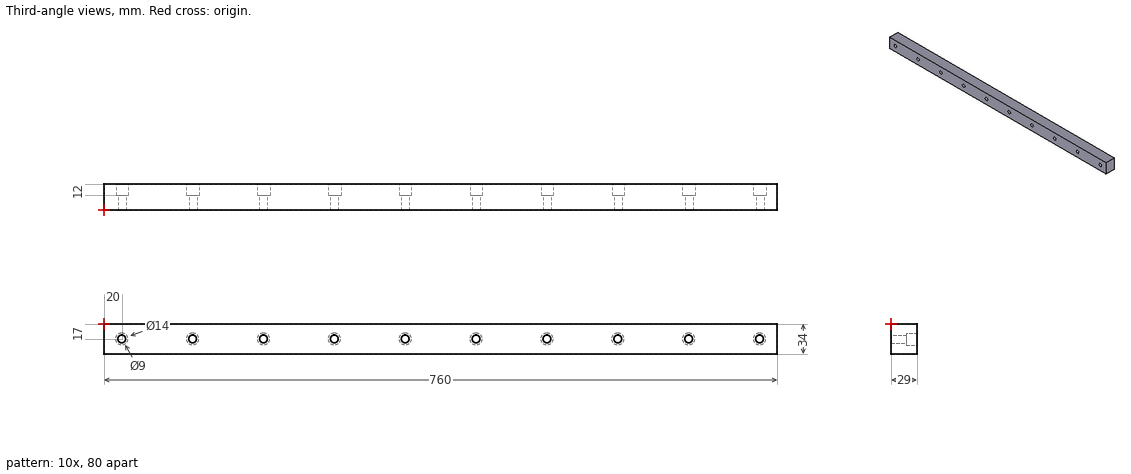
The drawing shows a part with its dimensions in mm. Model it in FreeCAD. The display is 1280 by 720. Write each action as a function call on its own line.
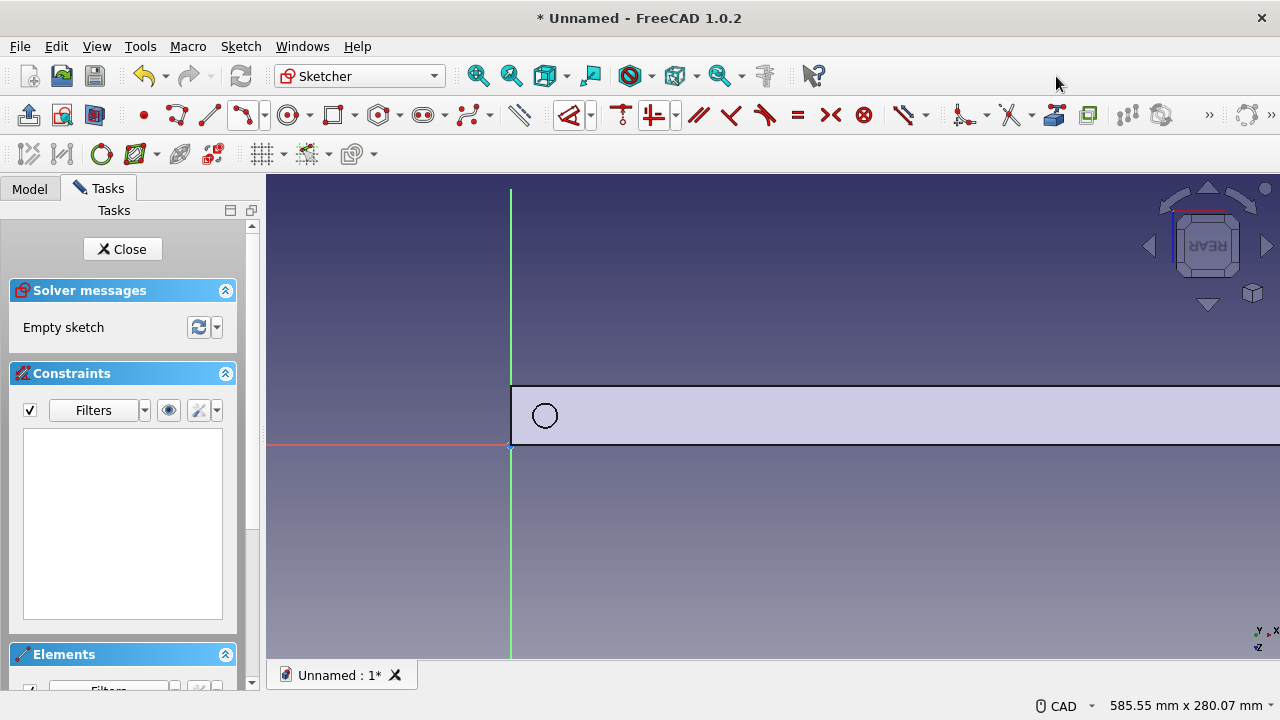
scroll(537, 416, up, 15)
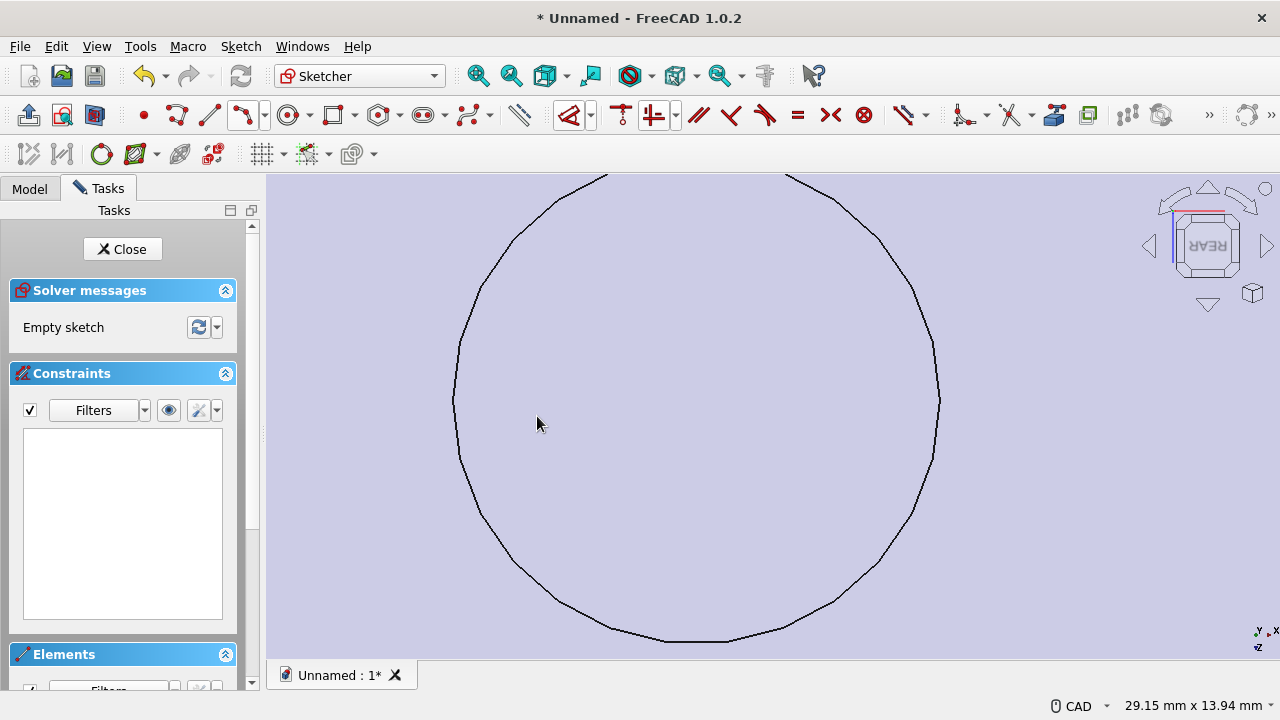
key(g)
key(c)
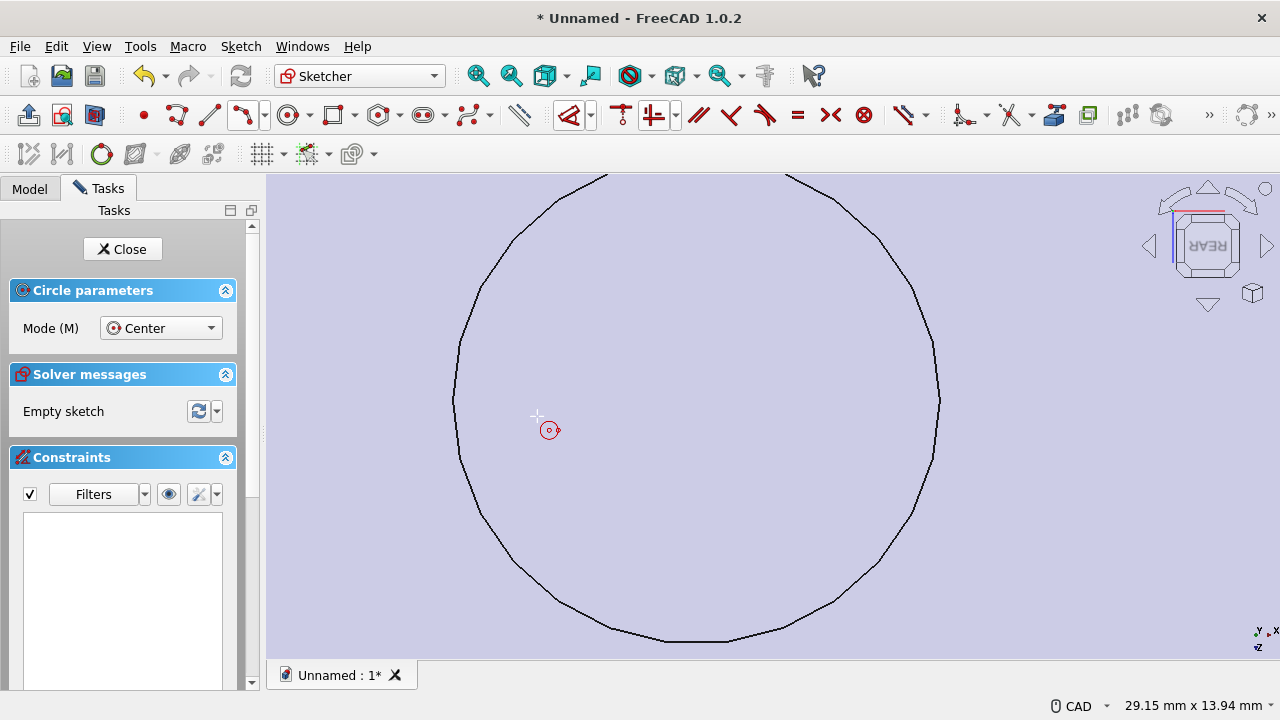
click(696, 400)
move(807, 290)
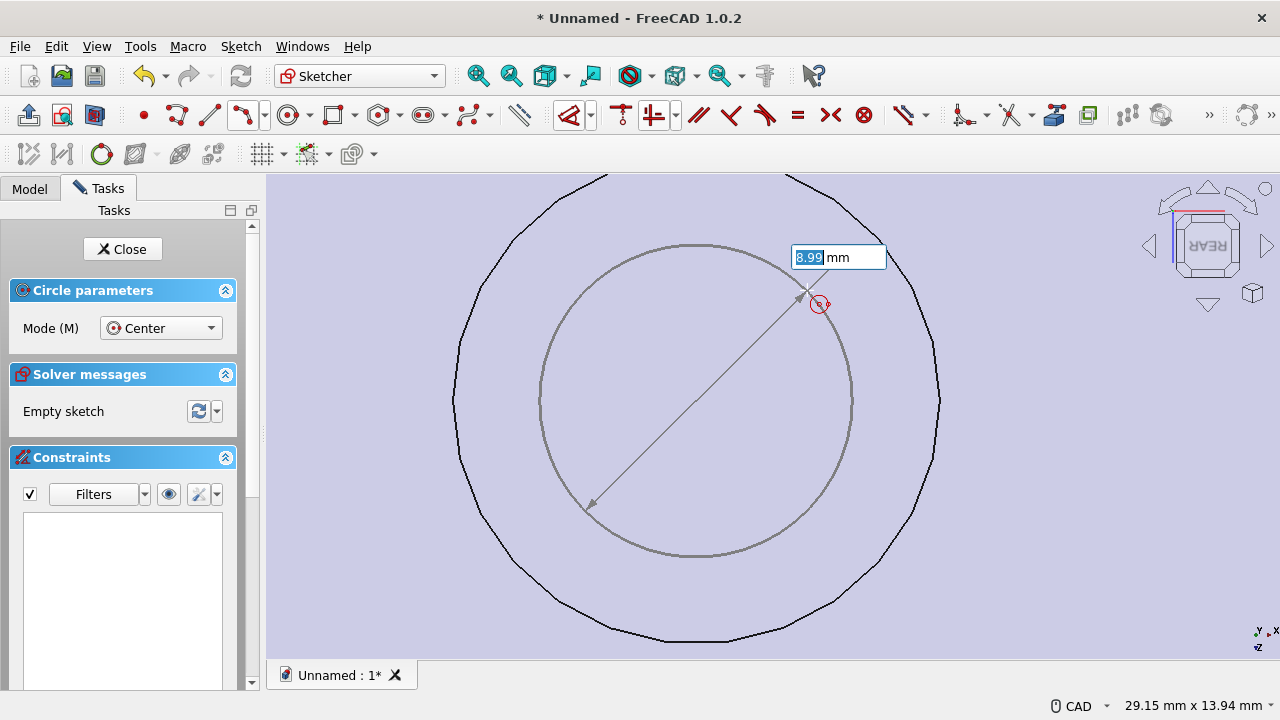
text(9)
key(Return)
key(Escape)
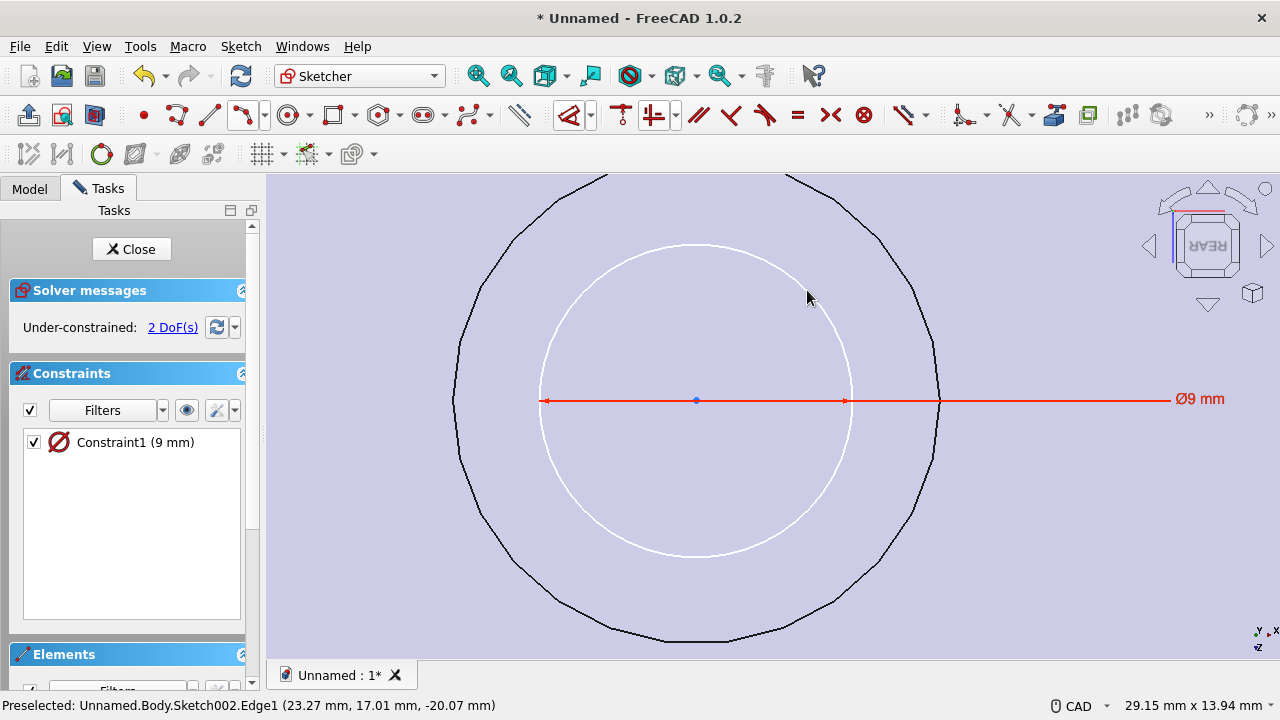
key(d)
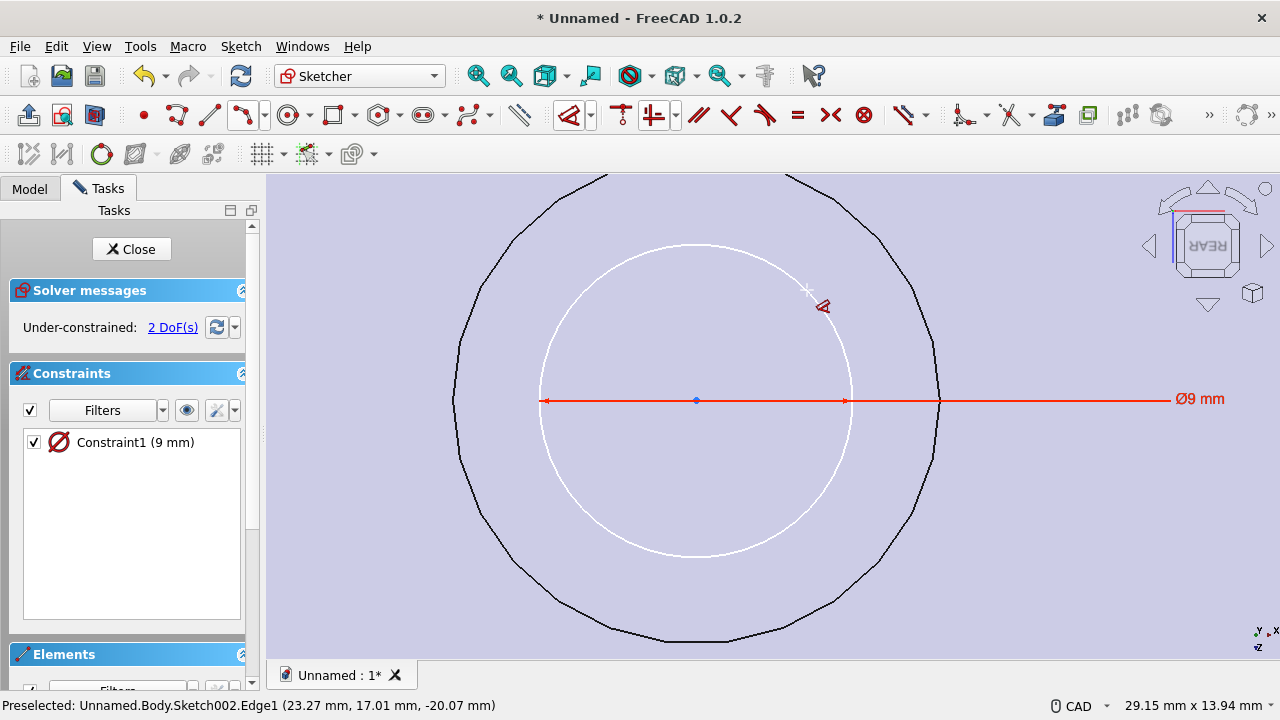
click(696, 401)
click(495, 367)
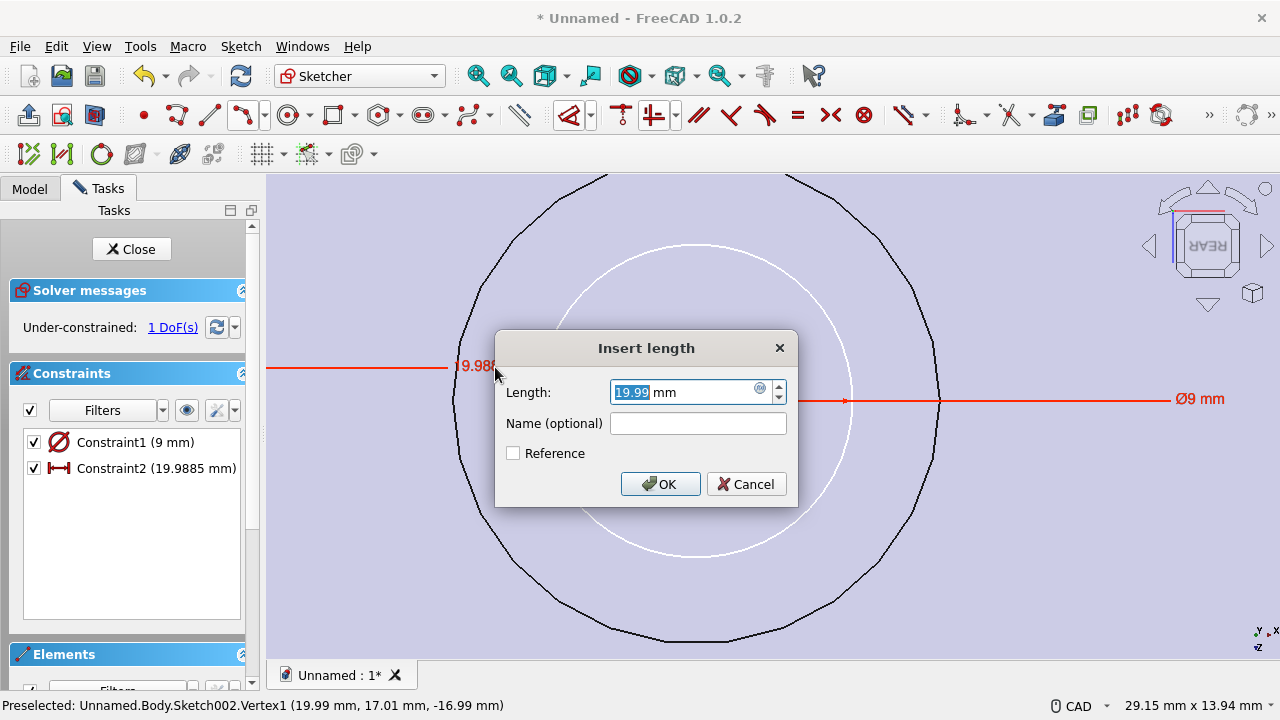
text(20)
key(Return)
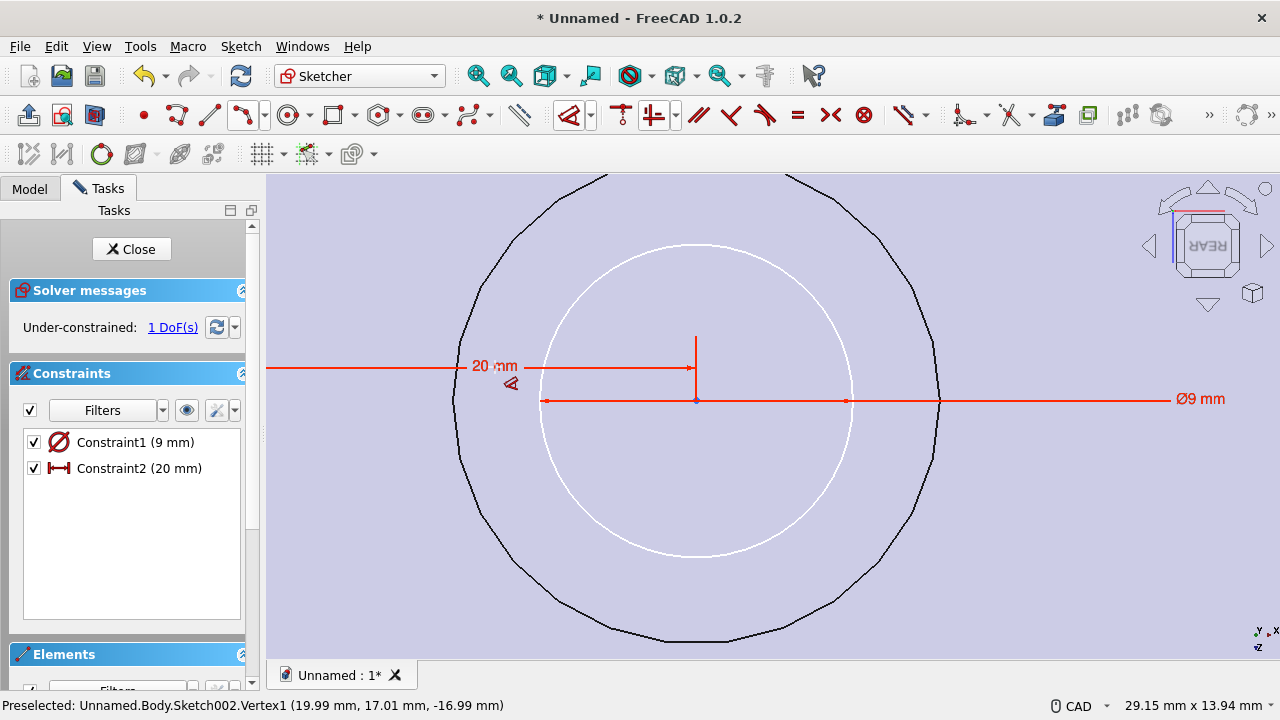
click(696, 401)
click(730, 516)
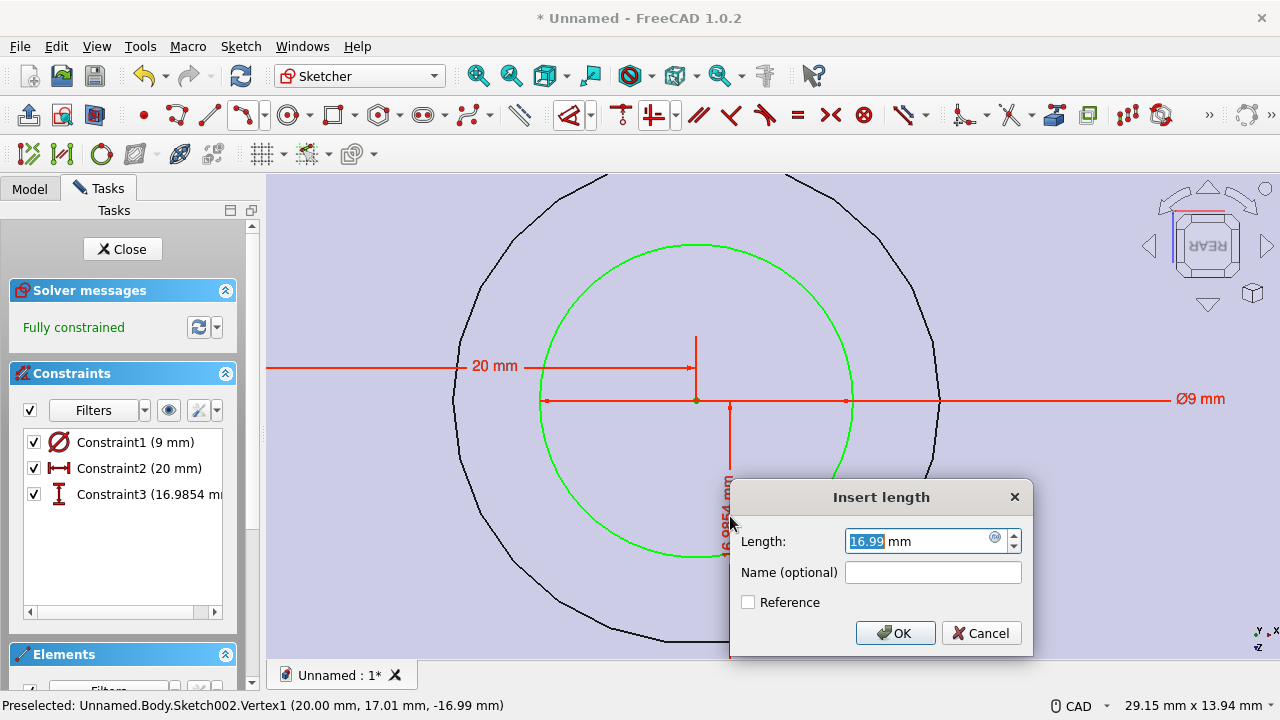
text(17)
key(Return)
key(Escape)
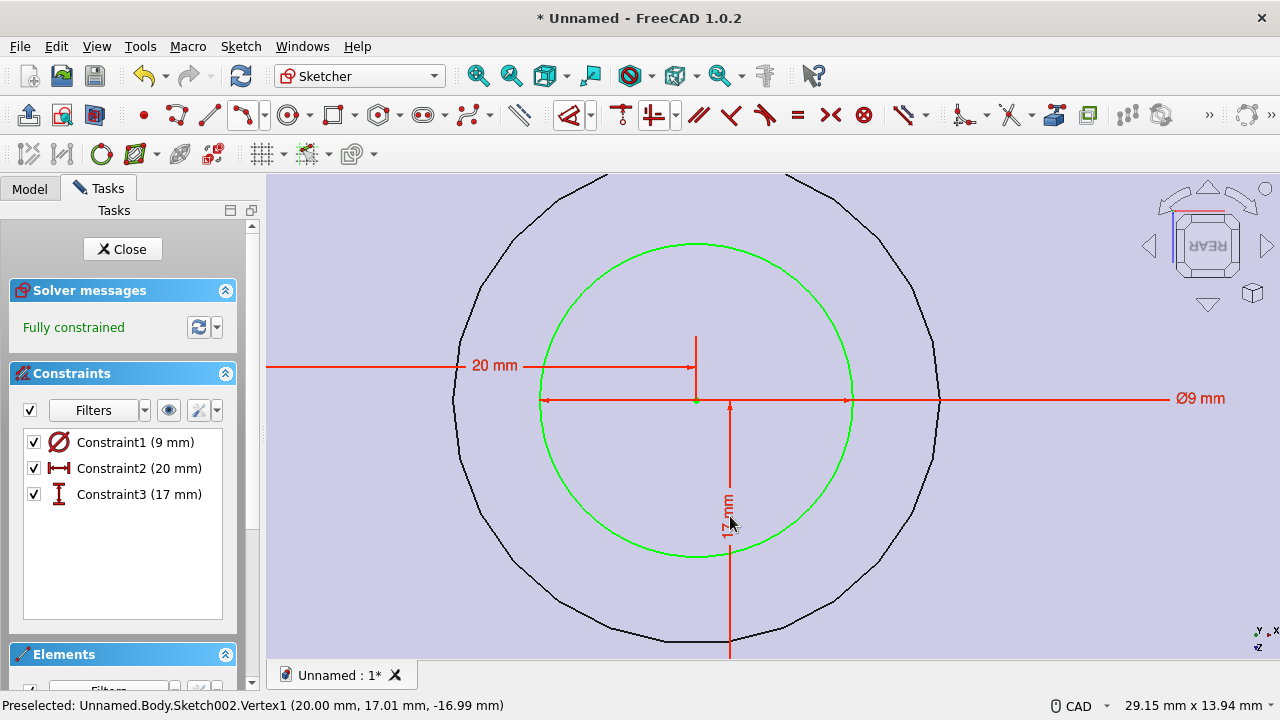
click(123, 249)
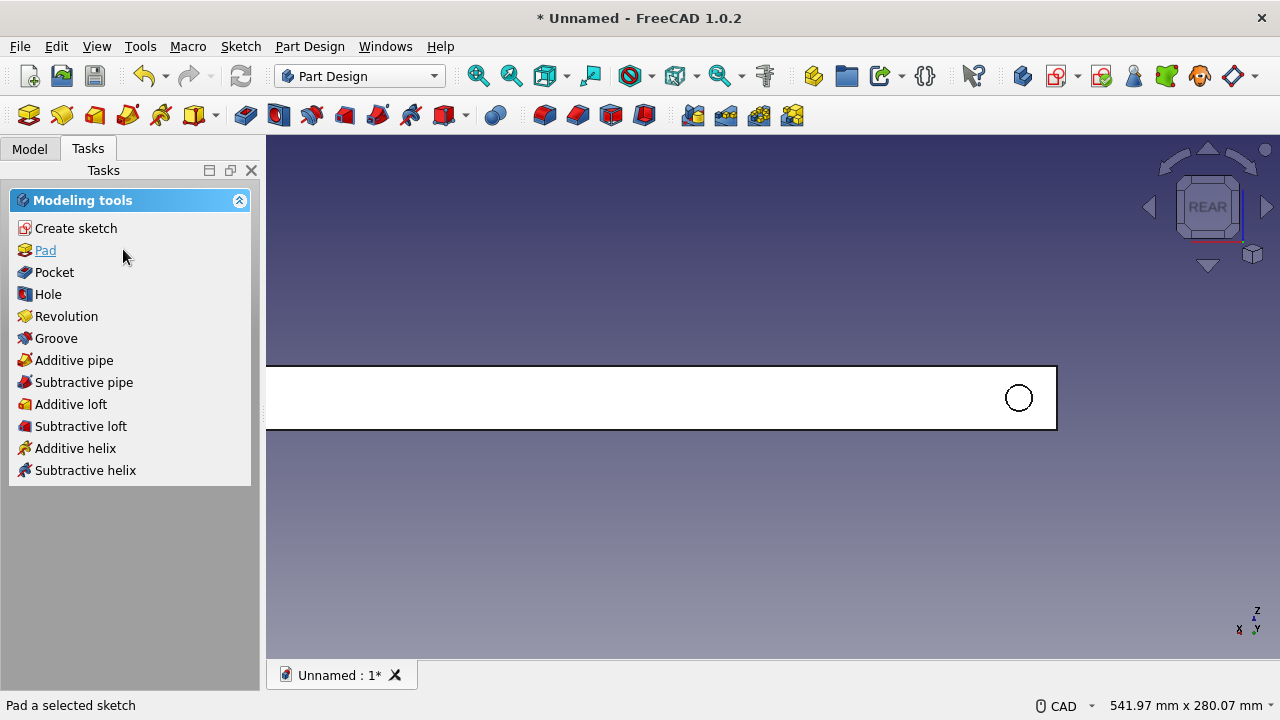
click(246, 116)